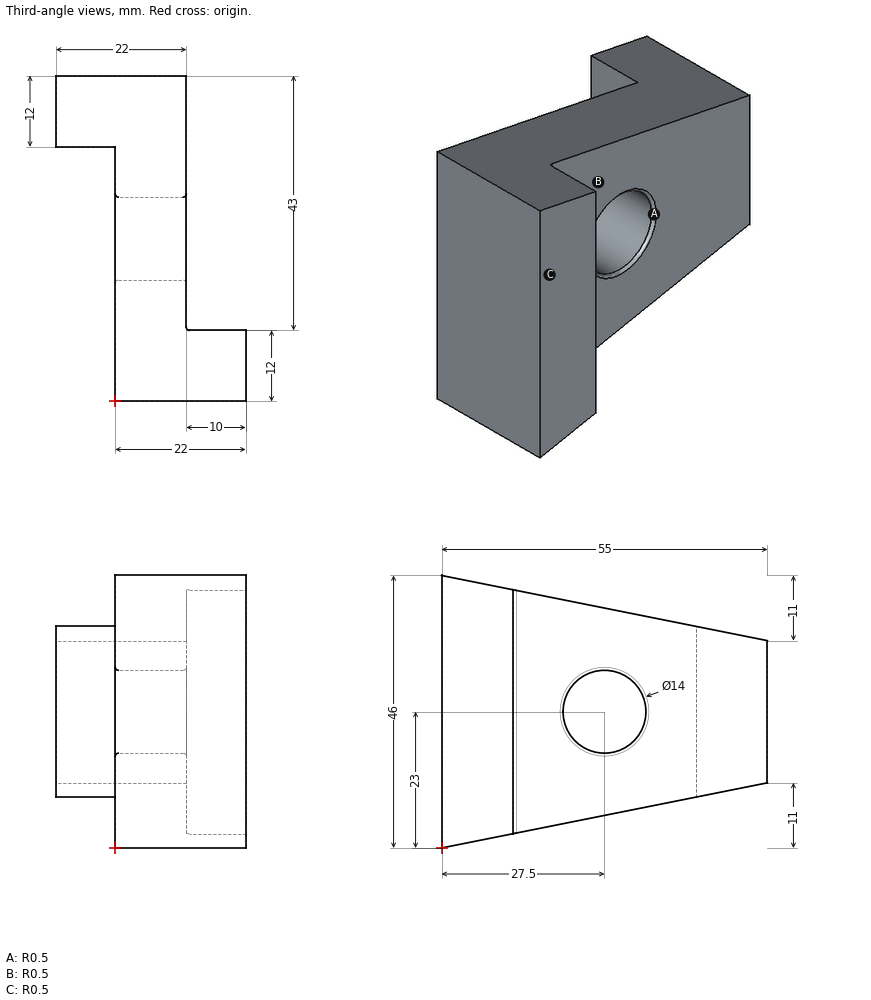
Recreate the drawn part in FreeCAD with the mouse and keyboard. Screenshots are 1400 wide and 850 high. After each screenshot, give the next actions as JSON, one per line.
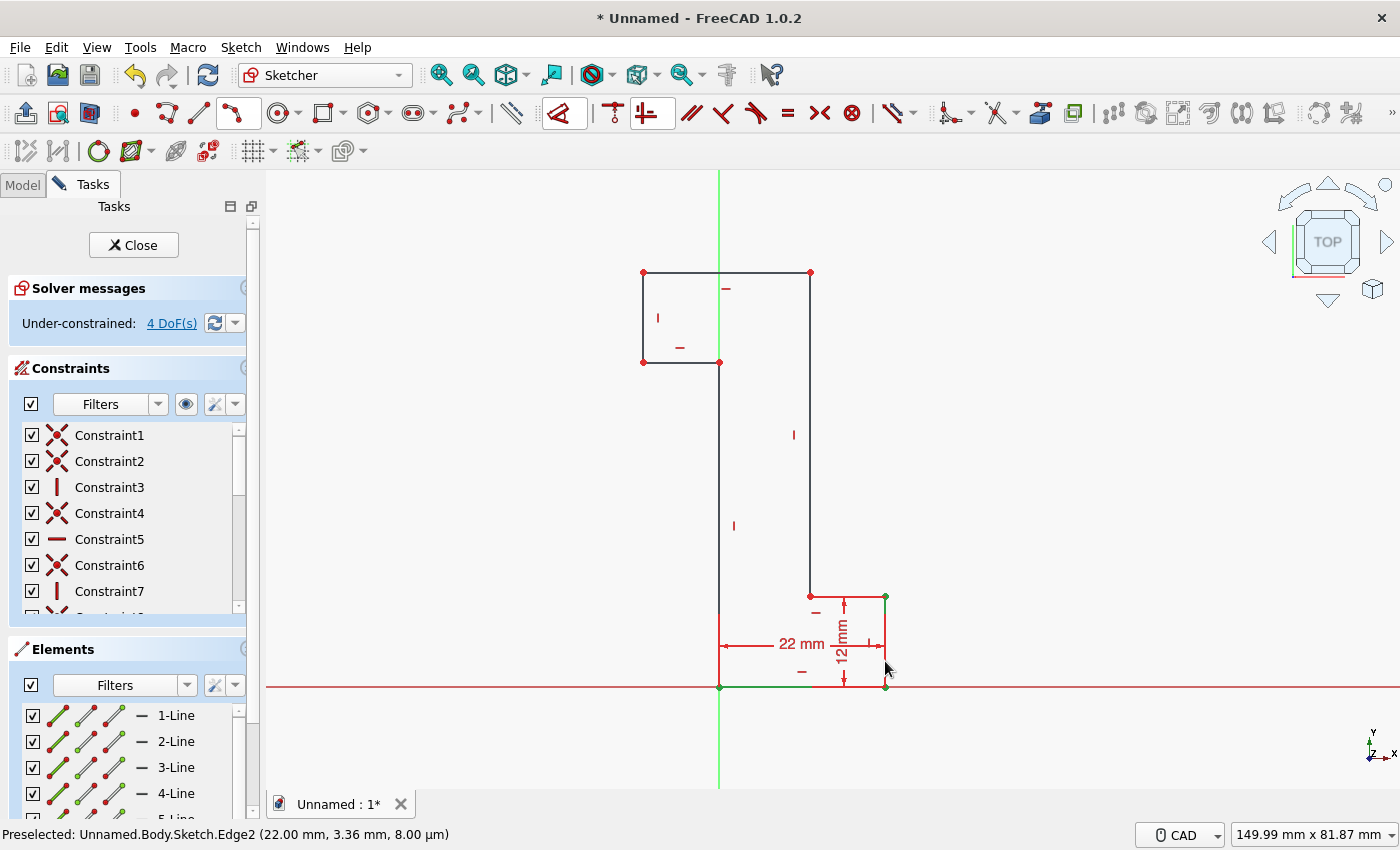
{"action": "left_click", "coordinate": [863, 597]}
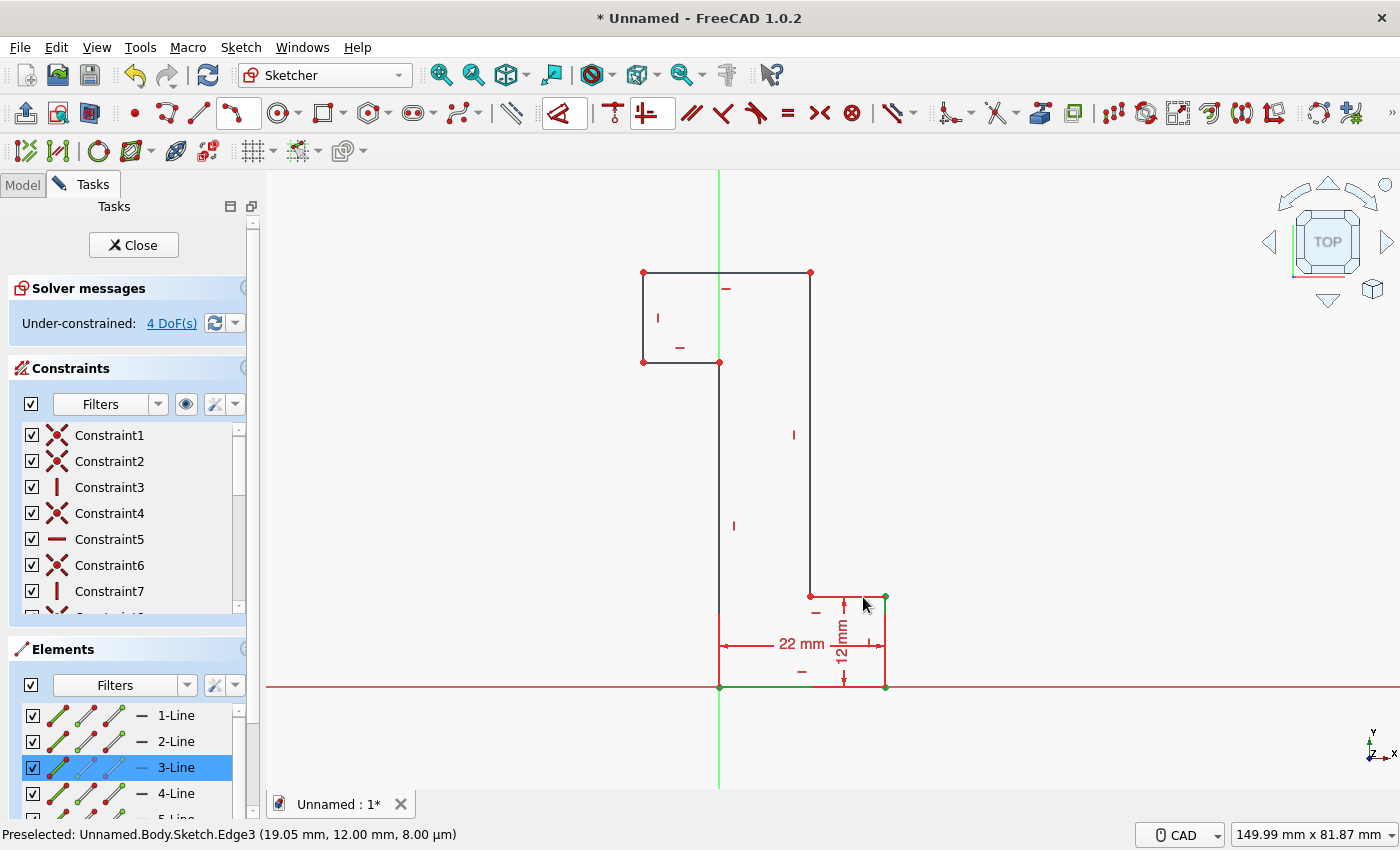
{"action": "left_click", "coordinate": [582, 114]}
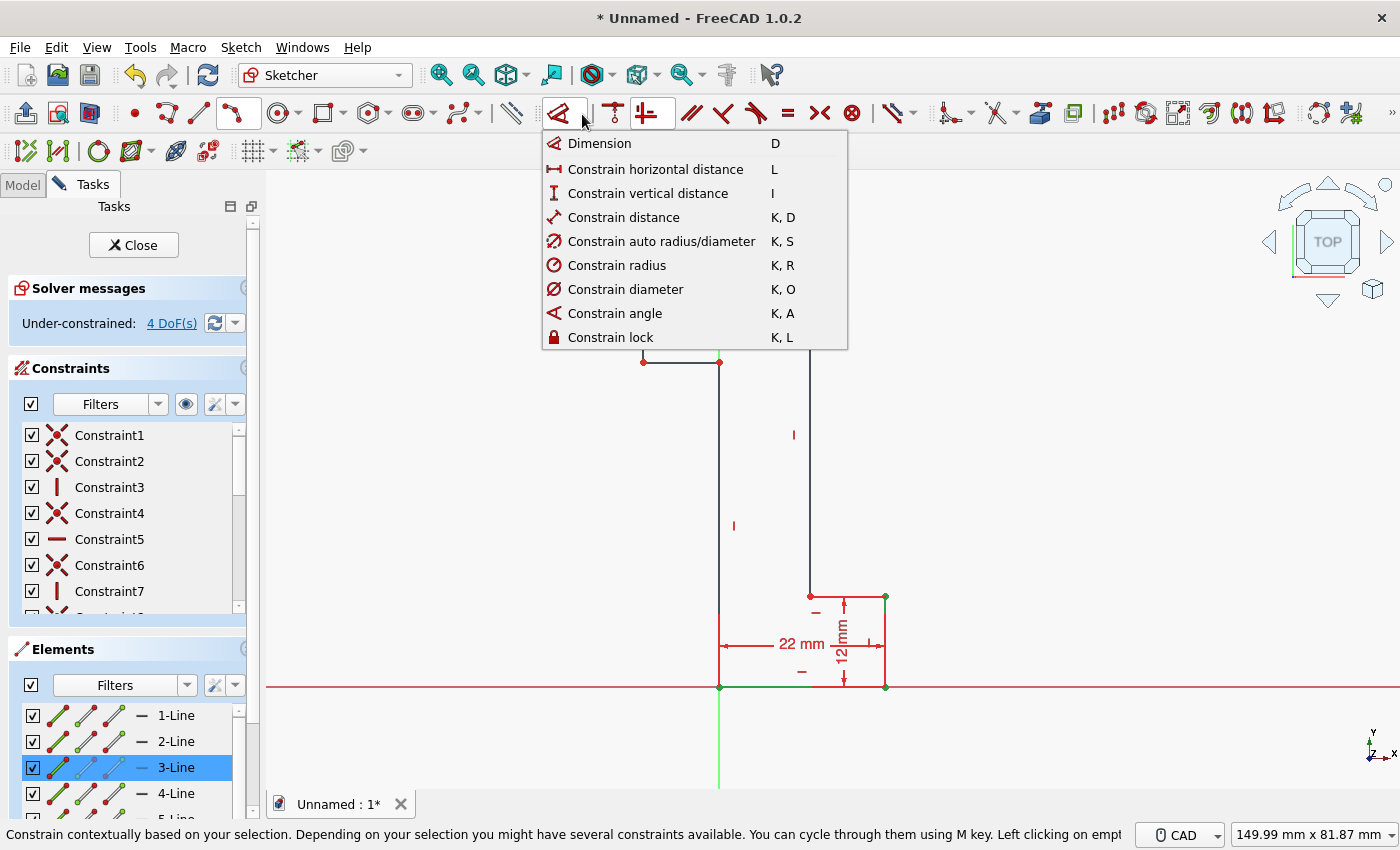
{"action": "left_click", "coordinate": [695, 169]}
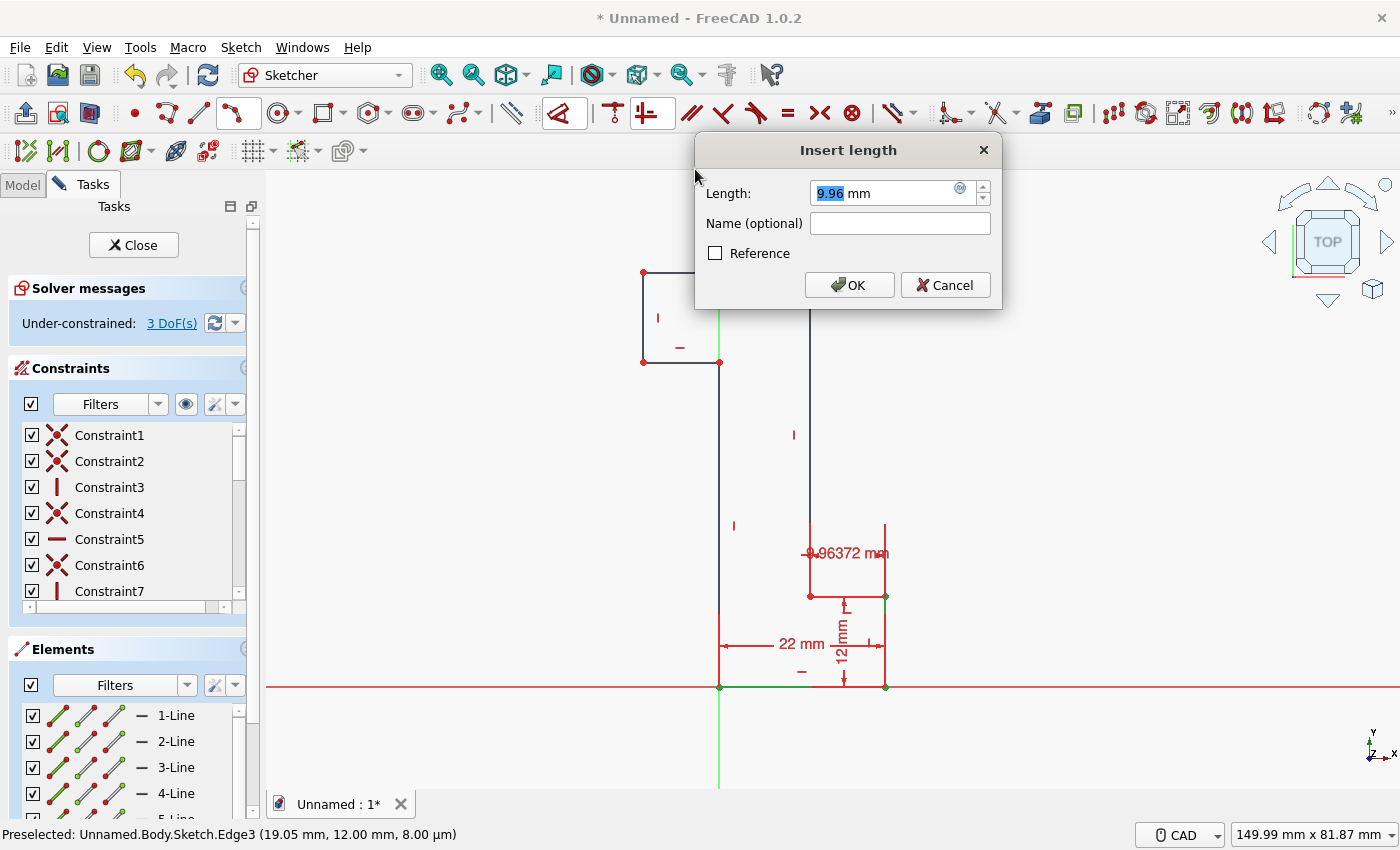
{"action": "type", "text": "10"}
{"action": "key", "text": "Return"}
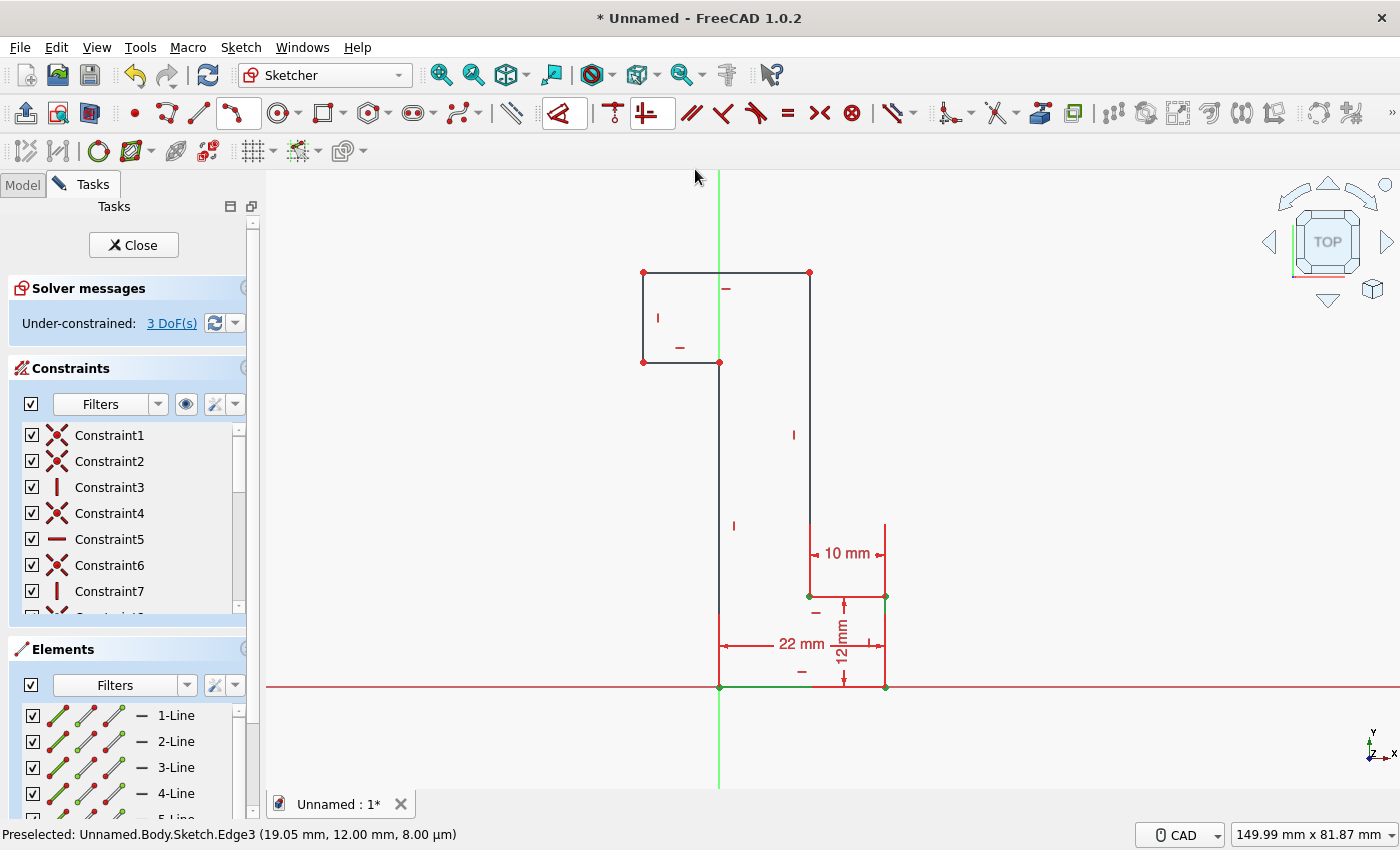
{"action": "left_click", "coordinate": [810, 500]}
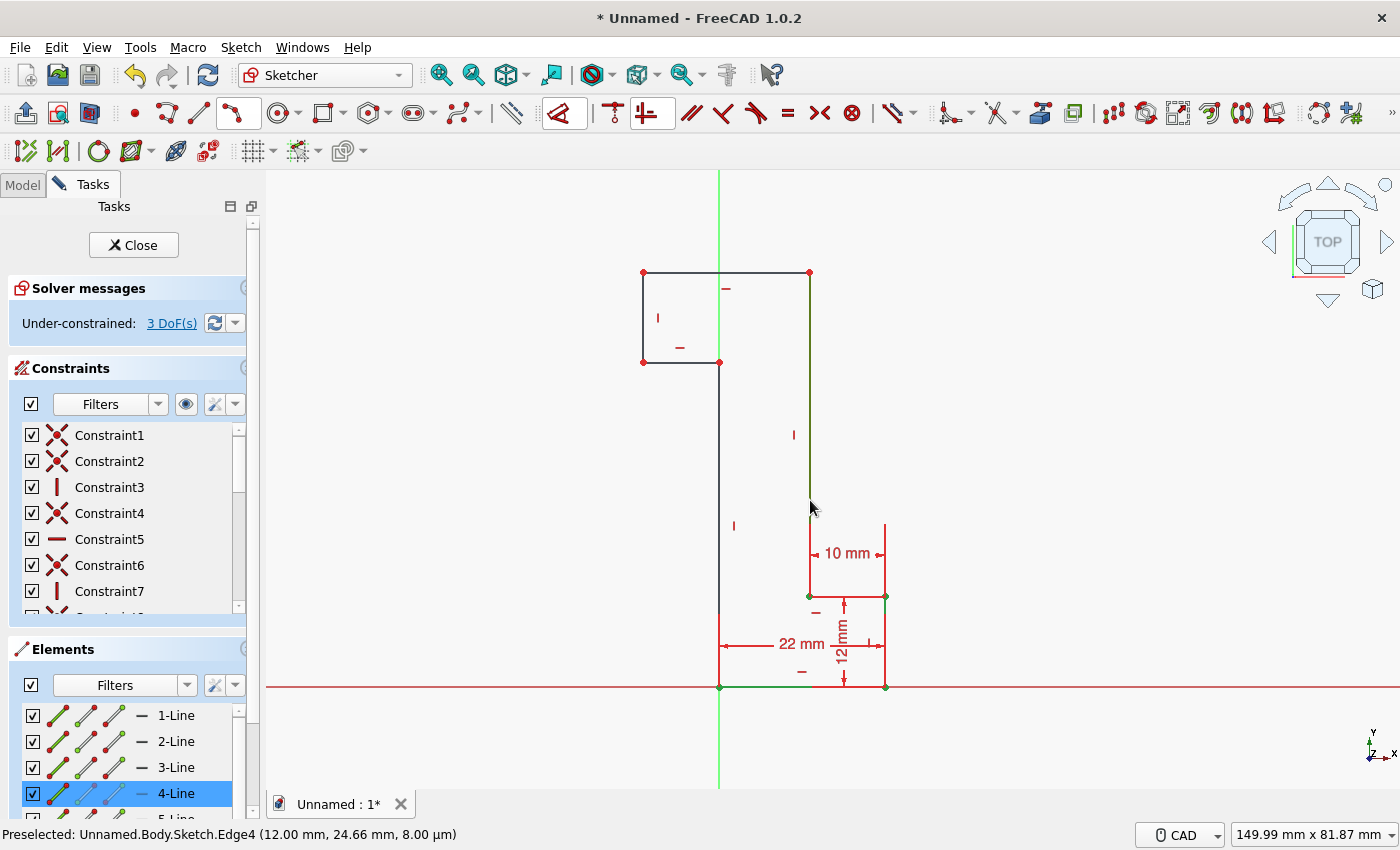
{"action": "left_click", "coordinate": [582, 114]}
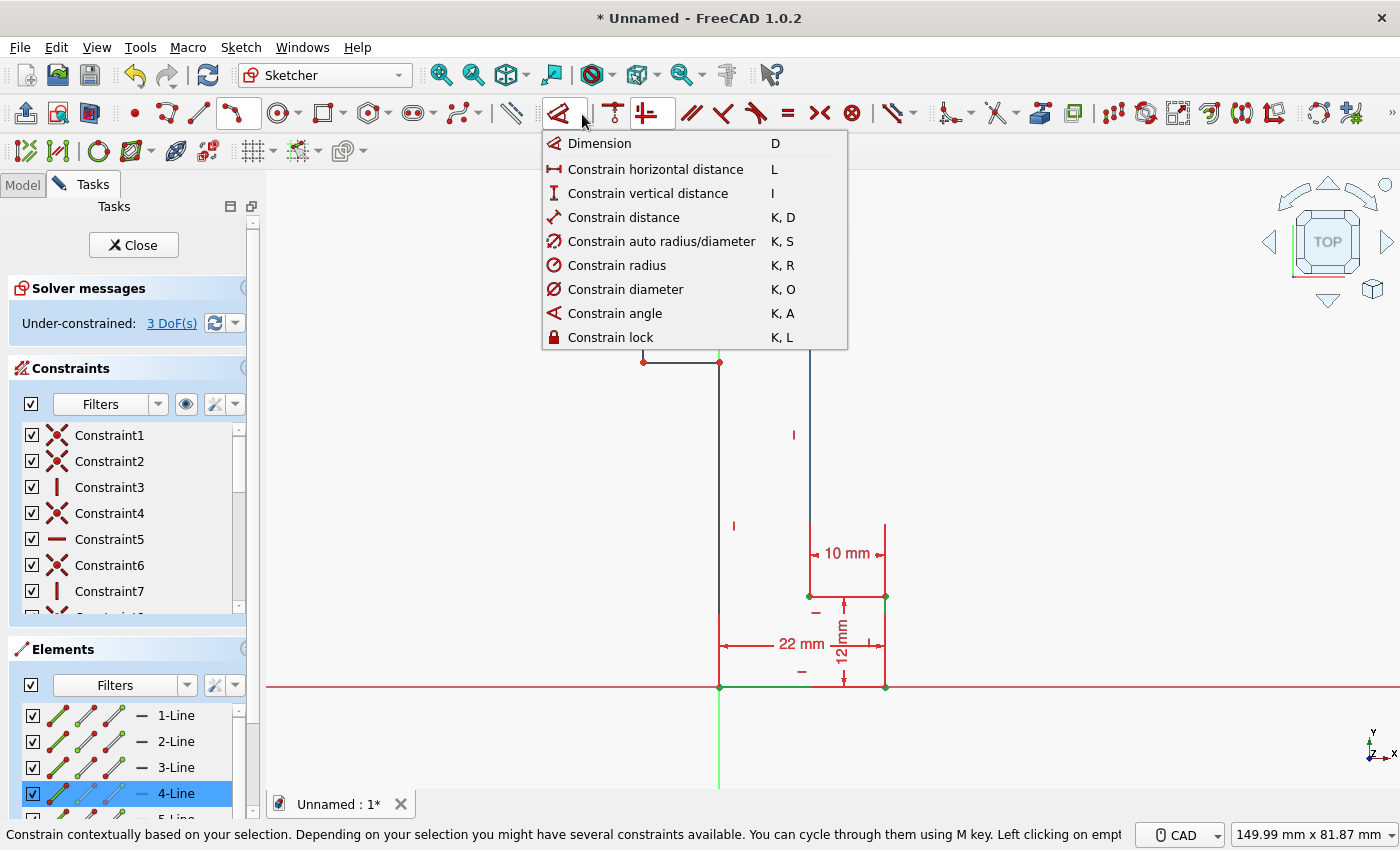
{"action": "left_click", "coordinate": [695, 193]}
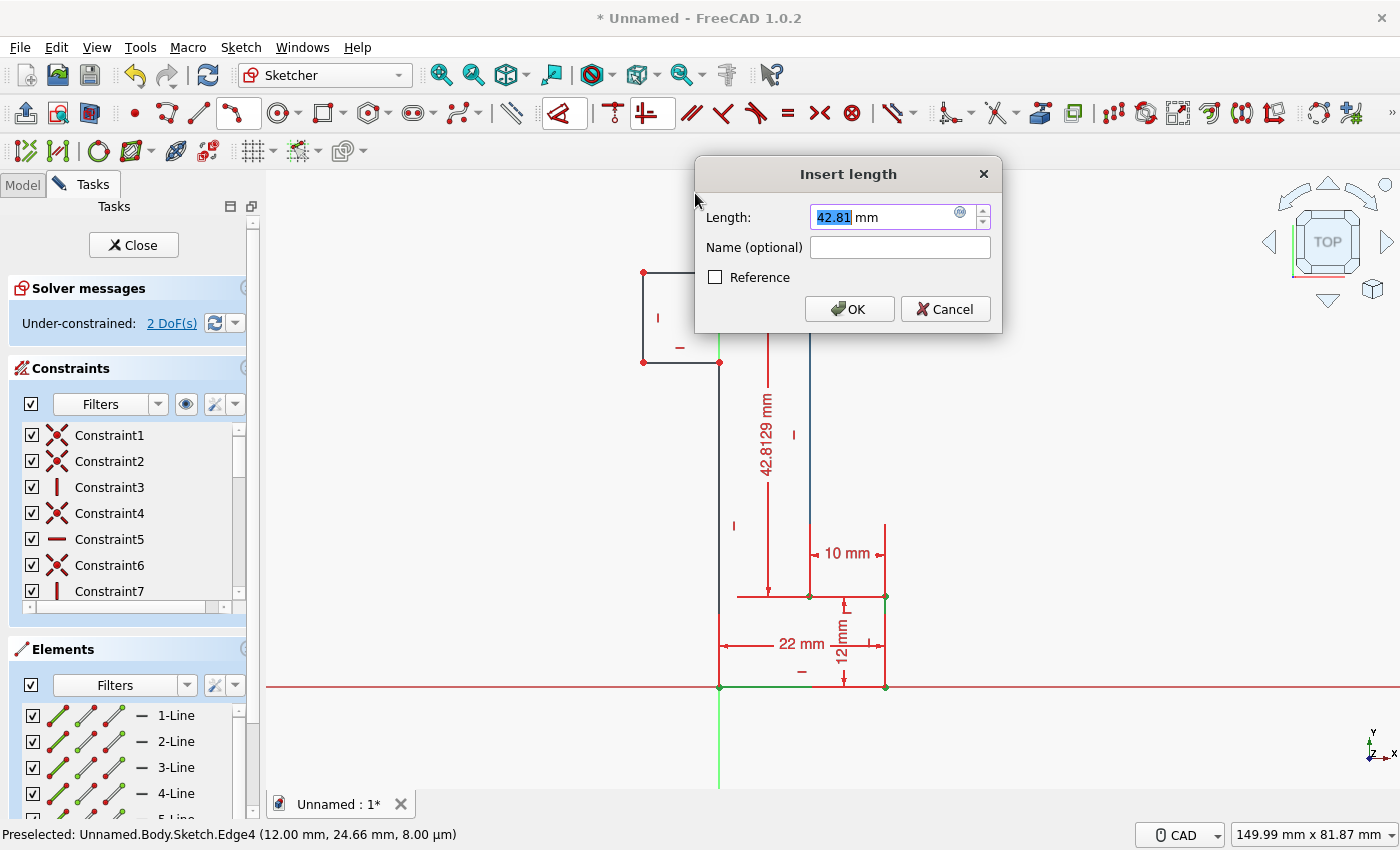
{"action": "type", "text": "43"}
{"action": "key", "text": "Return"}